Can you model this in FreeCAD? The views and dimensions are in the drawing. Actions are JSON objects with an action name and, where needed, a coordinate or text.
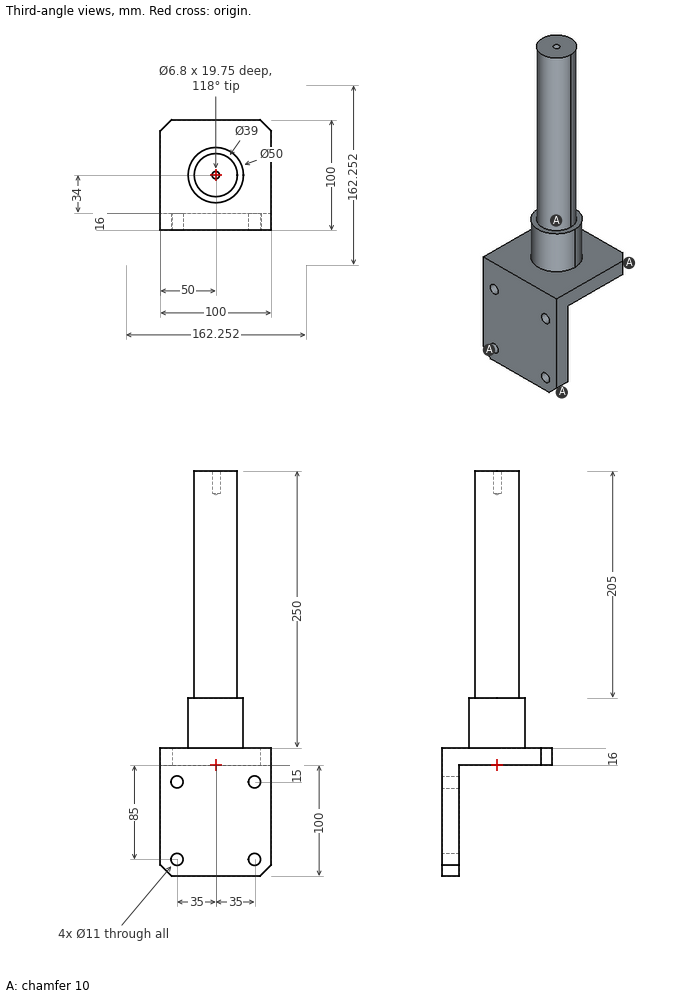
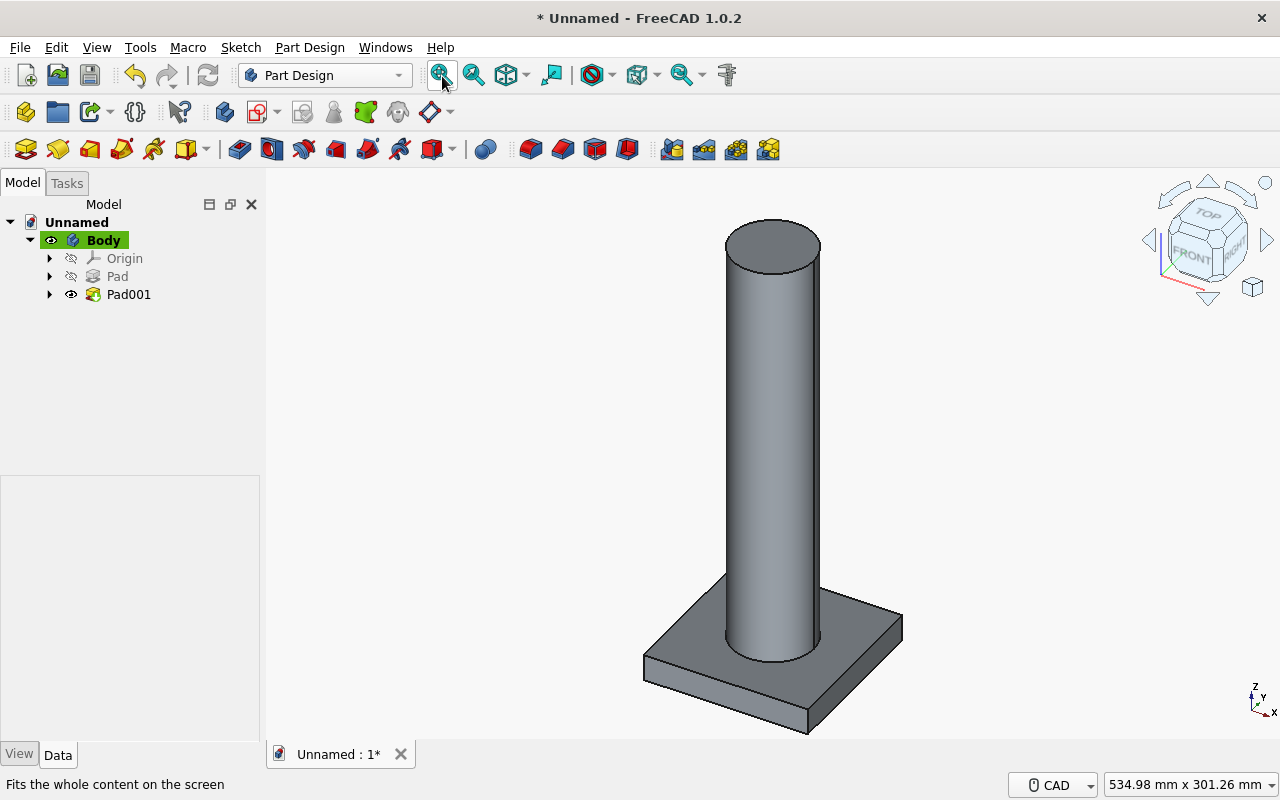
{"action": "left_click", "coordinate": [773, 246]}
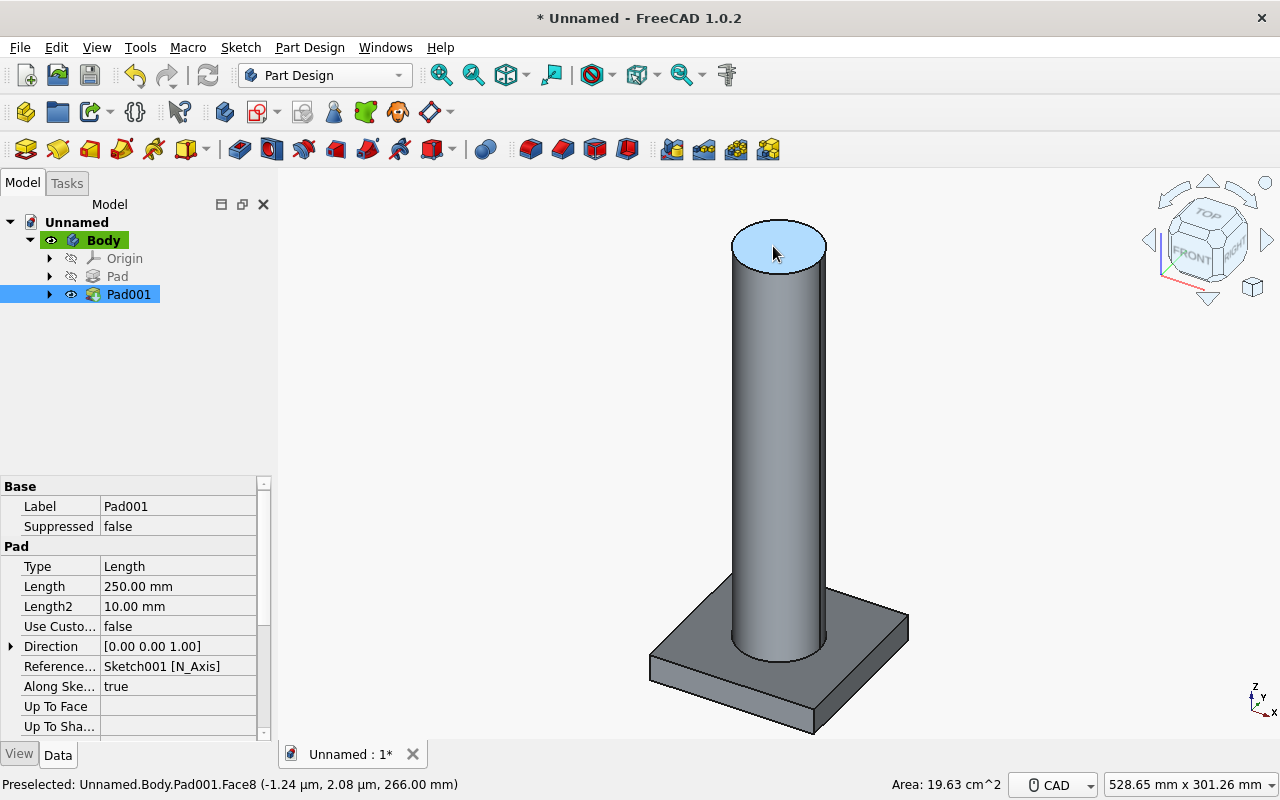
{"action": "left_click", "coordinate": [258, 112]}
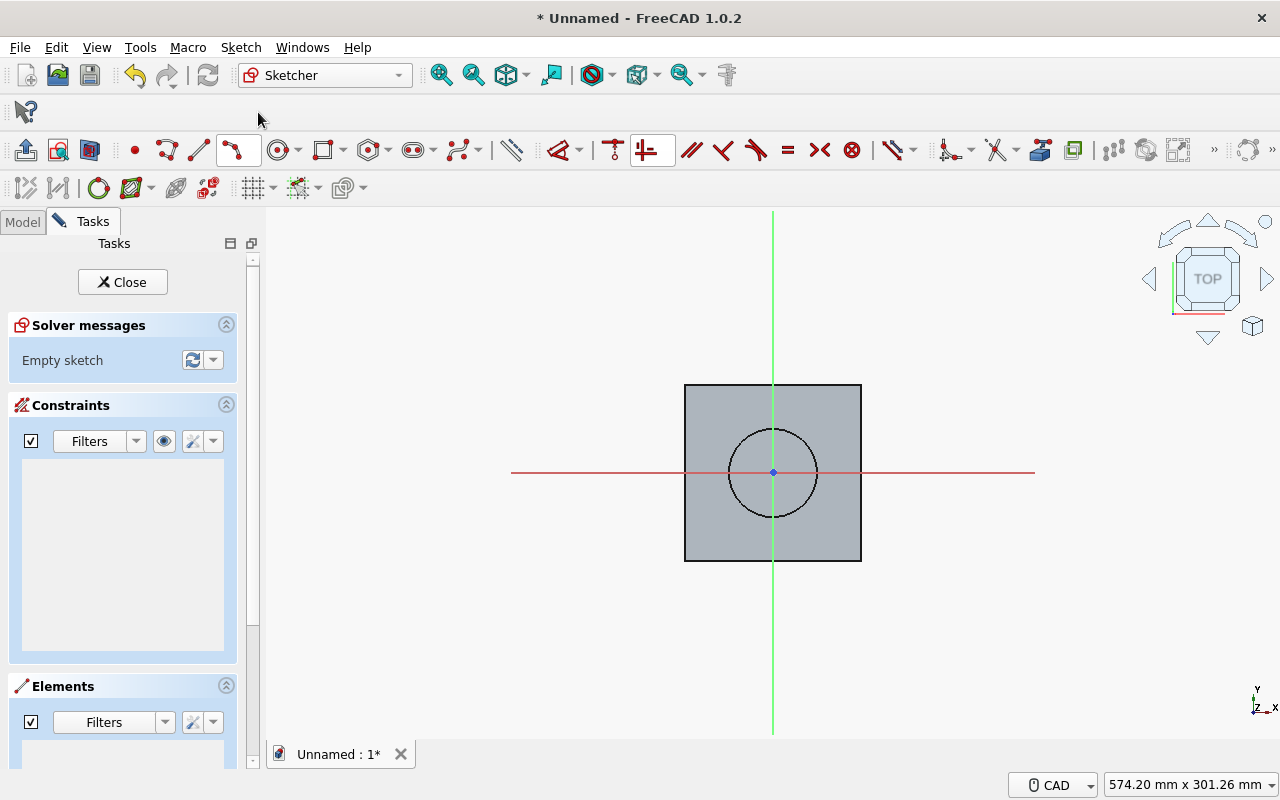
{"action": "key", "text": "g v"}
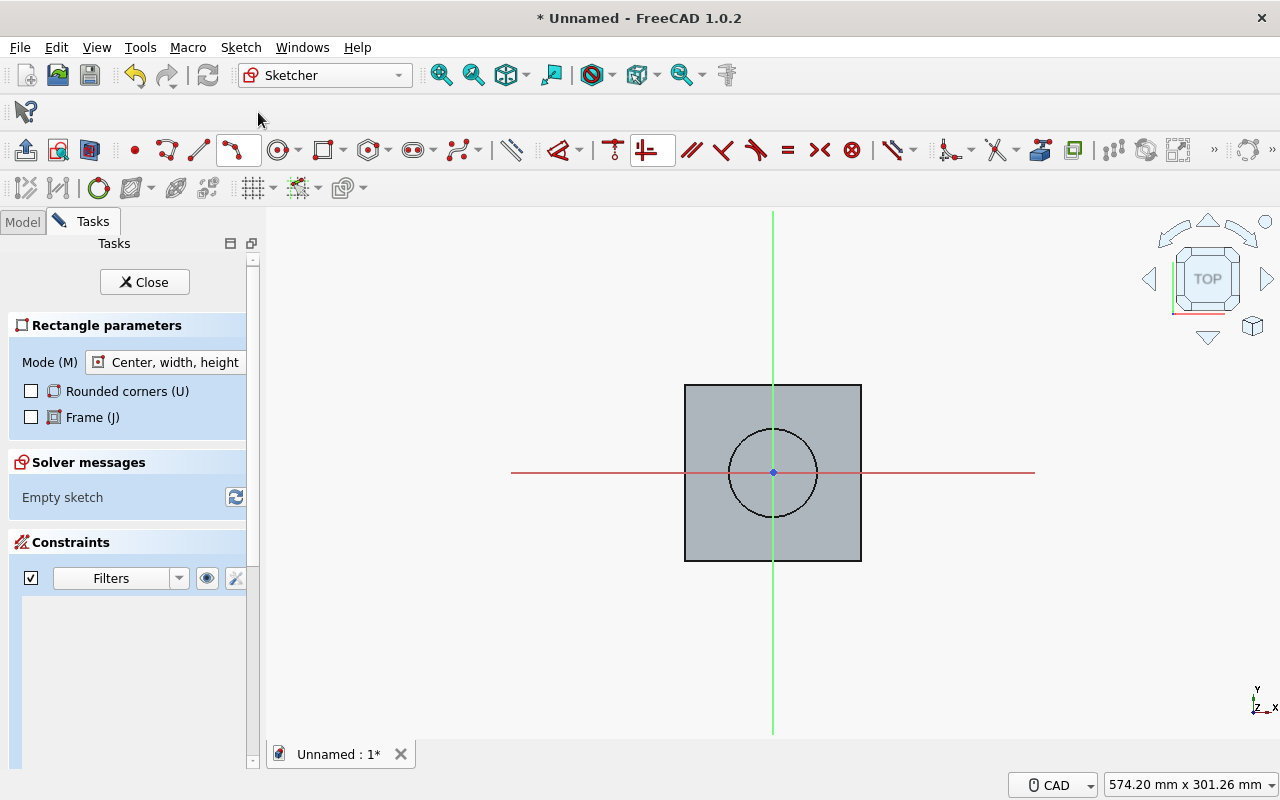
{"action": "left_click", "coordinate": [773, 473]}
{"action": "left_click", "coordinate": [916, 330]}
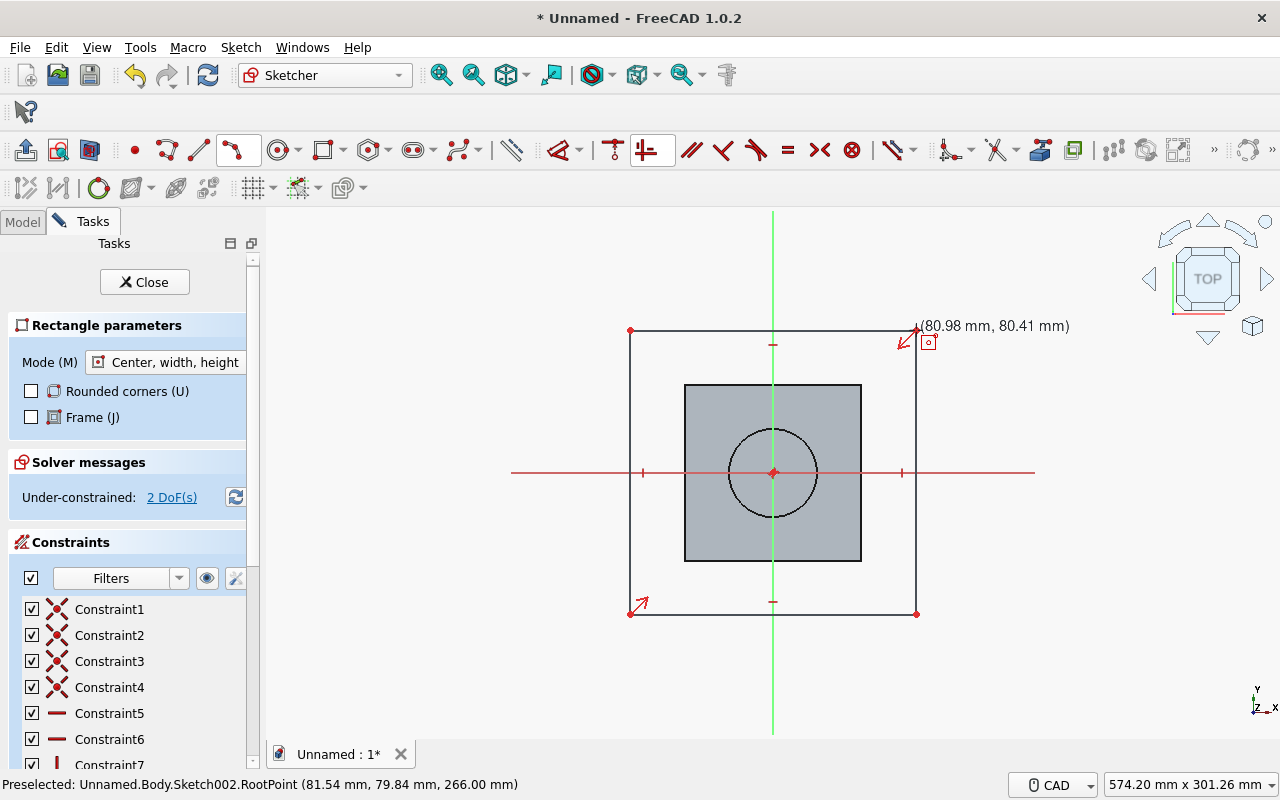
{"action": "key", "text": "g c"}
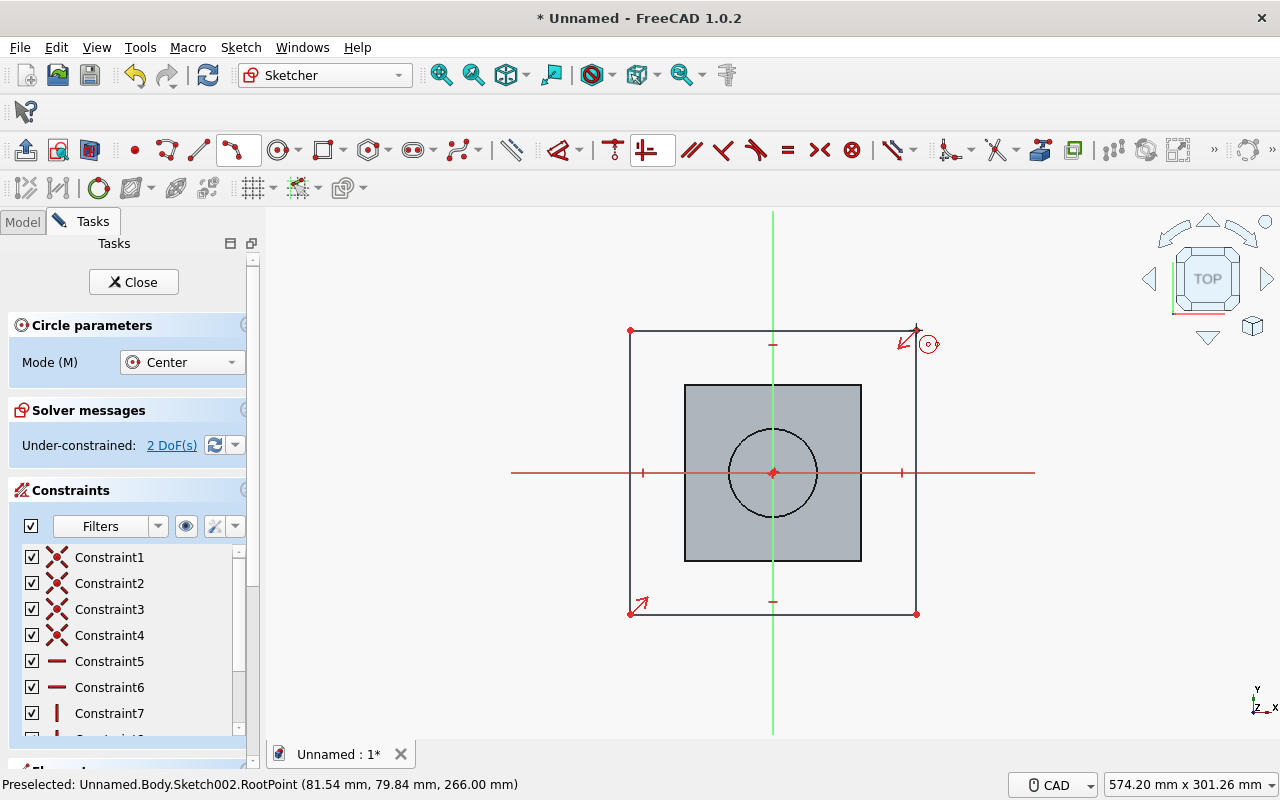
{"action": "left_click", "coordinate": [773, 473]}
{"action": "left_click", "coordinate": [797, 449]}
{"action": "key", "text": "Escape"}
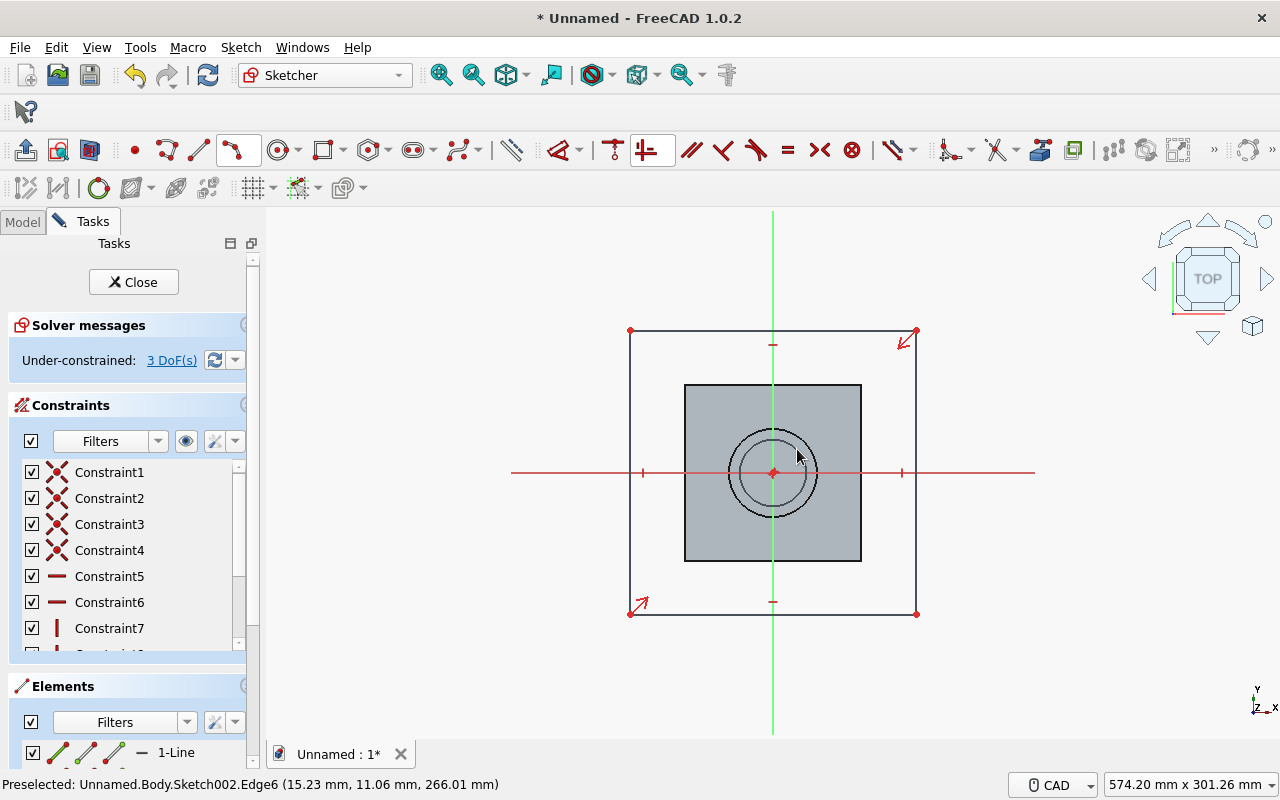
{"action": "left_click", "coordinate": [558, 150]}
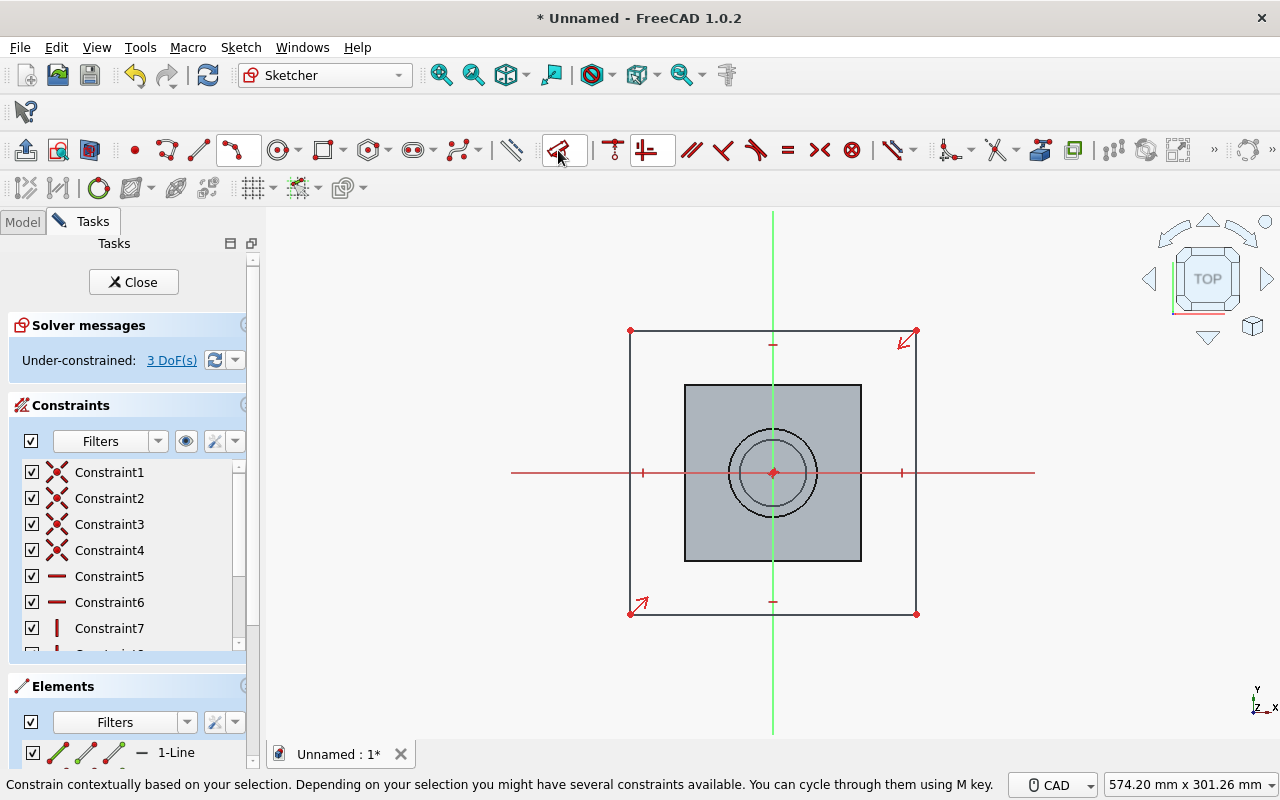
{"action": "left_click", "coordinate": [796, 449]}
{"action": "left_click", "coordinate": [818, 426]}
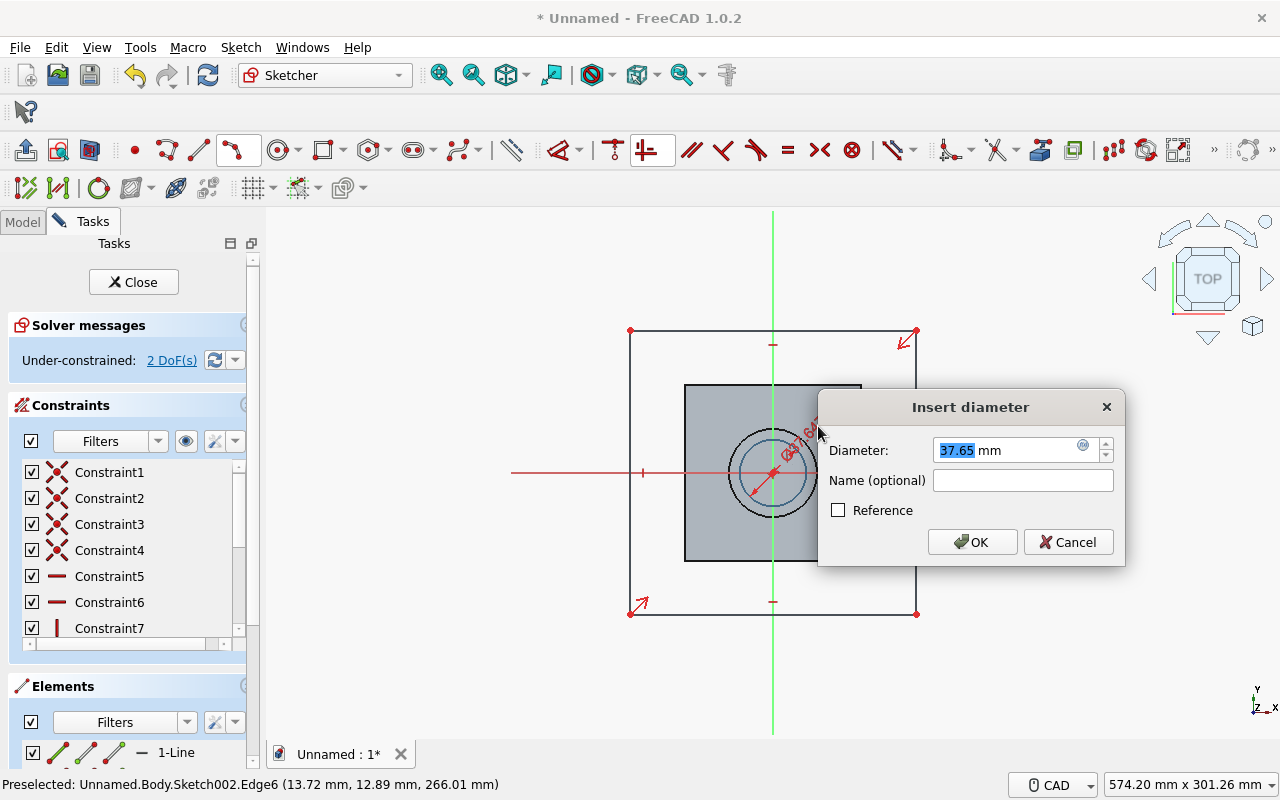
{"action": "type", "text": "39"}
{"action": "key", "text": "Return"}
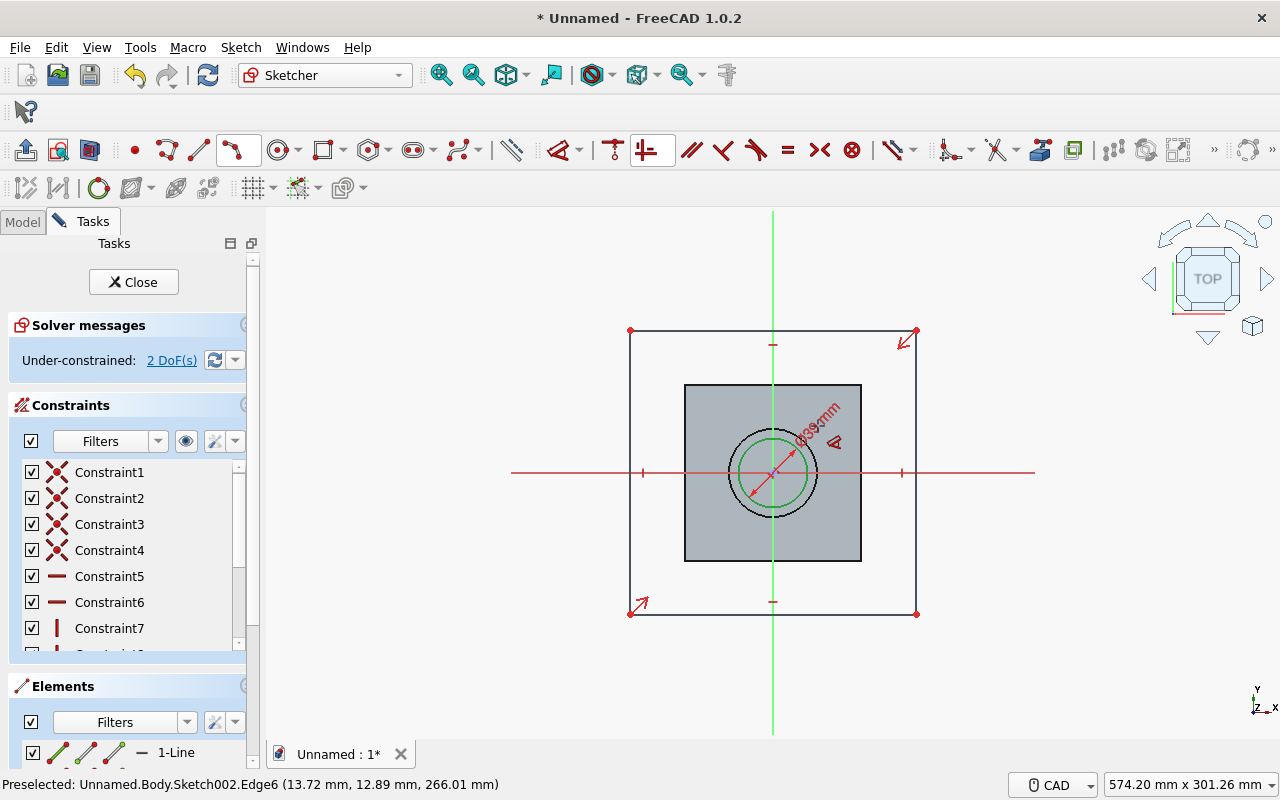
{"action": "left_click", "coordinate": [716, 615]}
{"action": "left_click", "coordinate": [707, 649]}